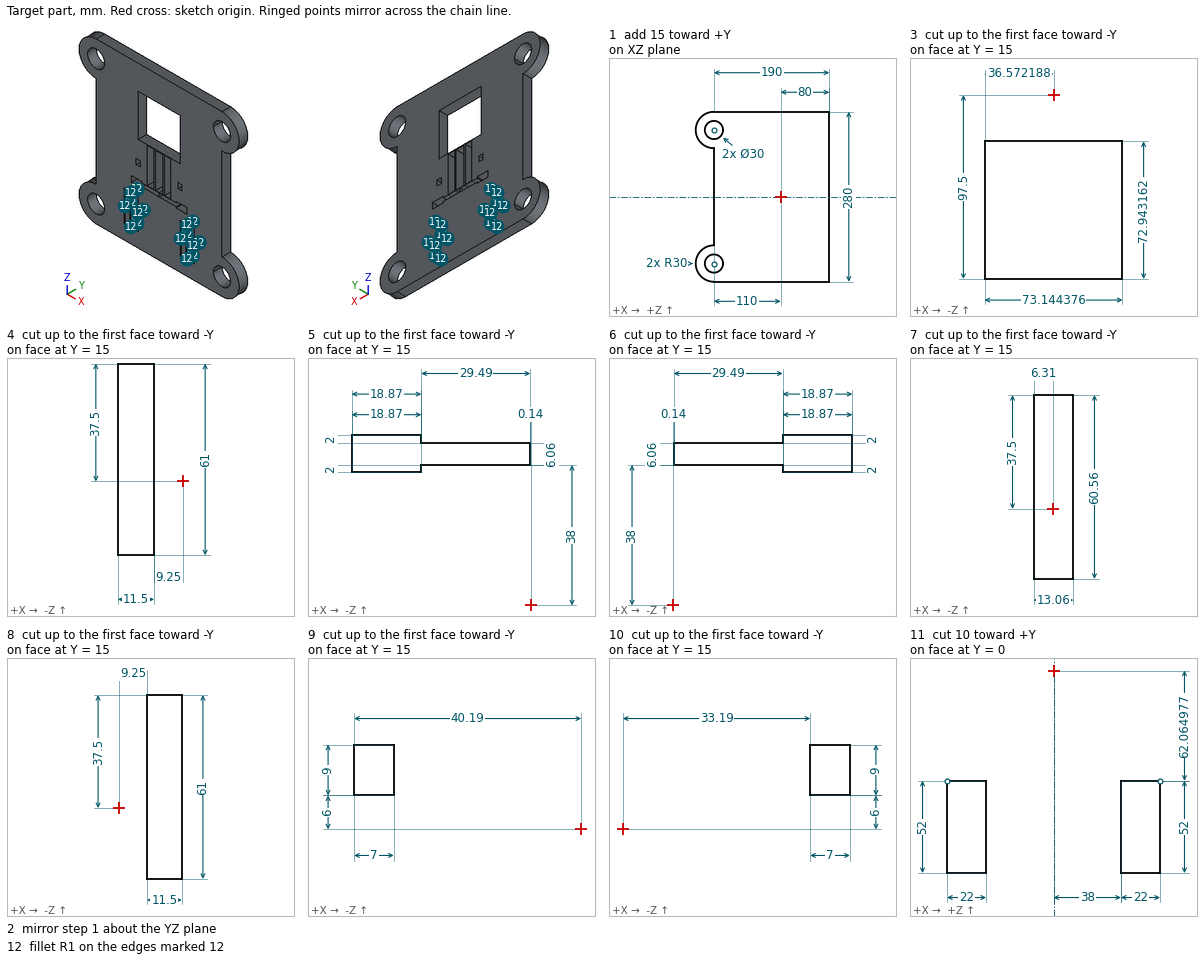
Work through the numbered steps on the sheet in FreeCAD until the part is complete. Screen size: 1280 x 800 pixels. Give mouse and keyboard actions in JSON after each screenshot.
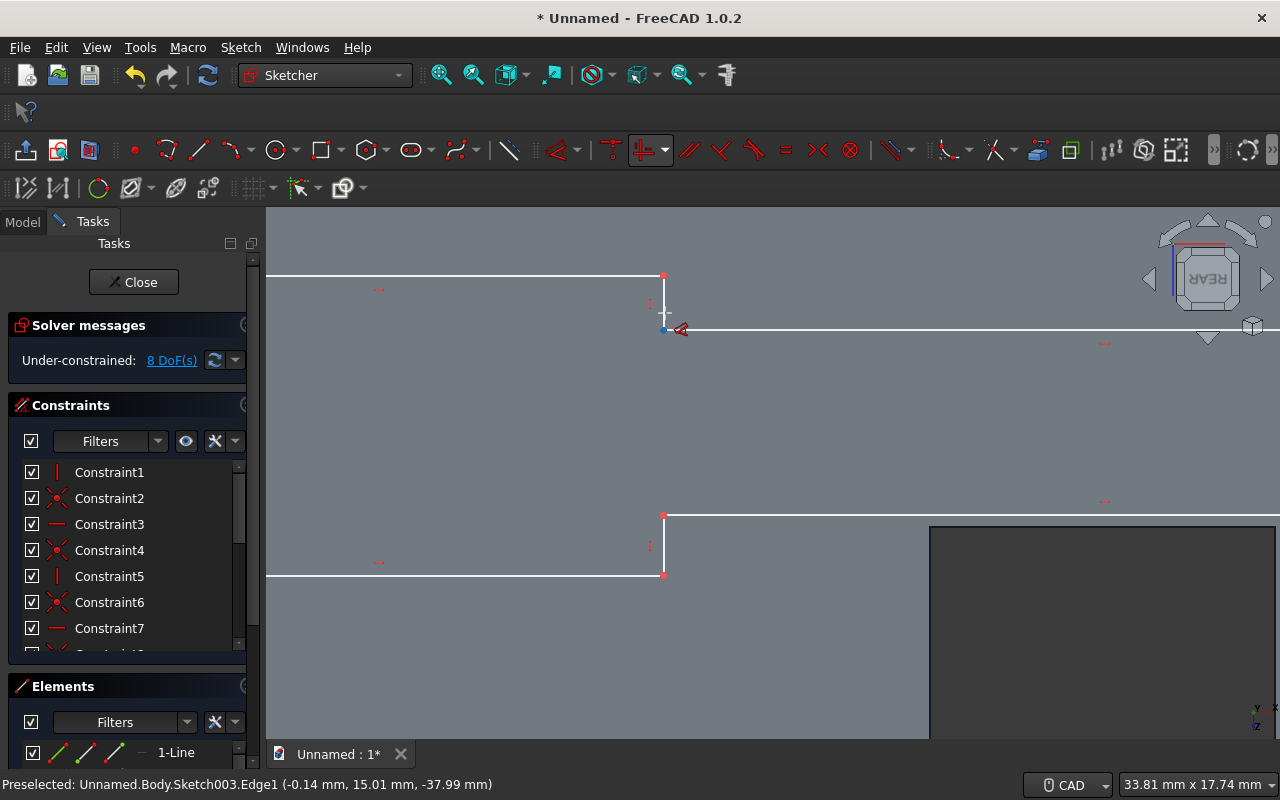
{"action": "left_click", "coordinate": [664, 314]}
{"action": "left_click", "coordinate": [630, 303]}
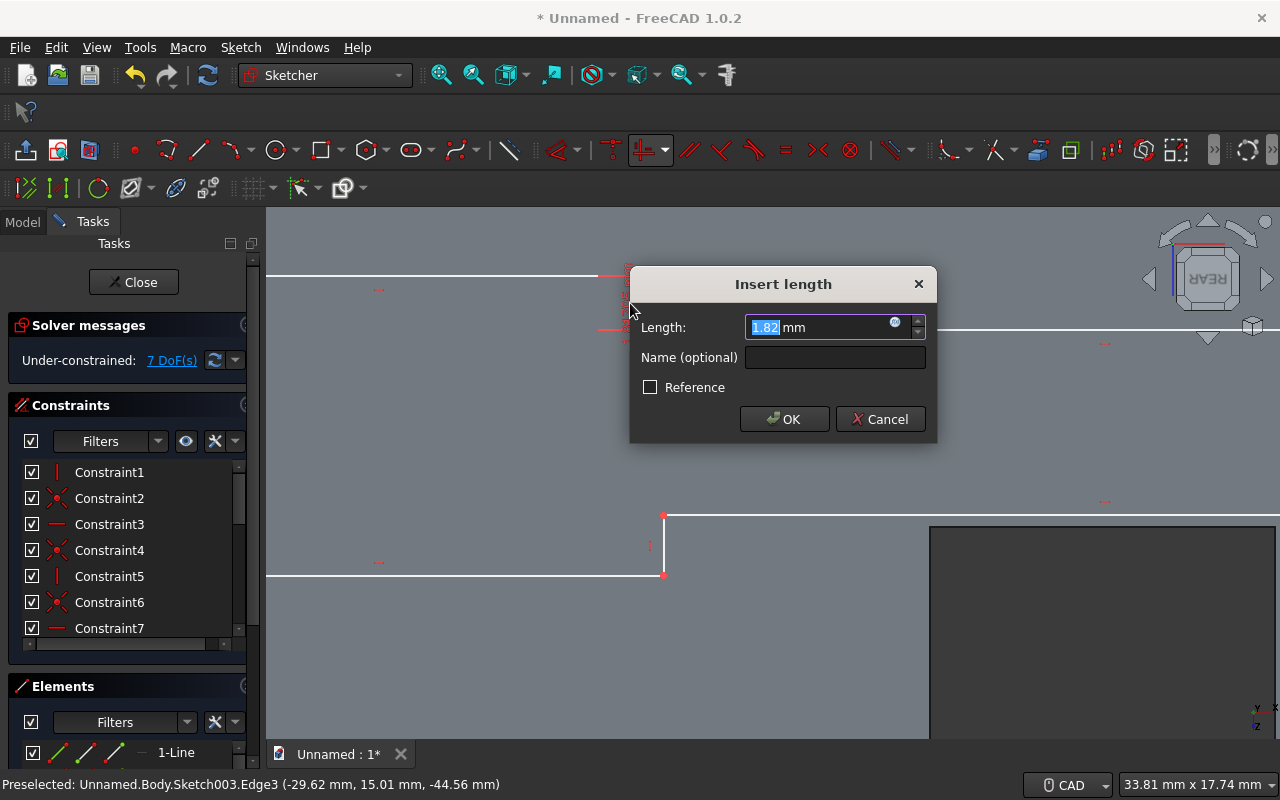
{"action": "type", "text": "2"}
{"action": "key", "text": "Return"}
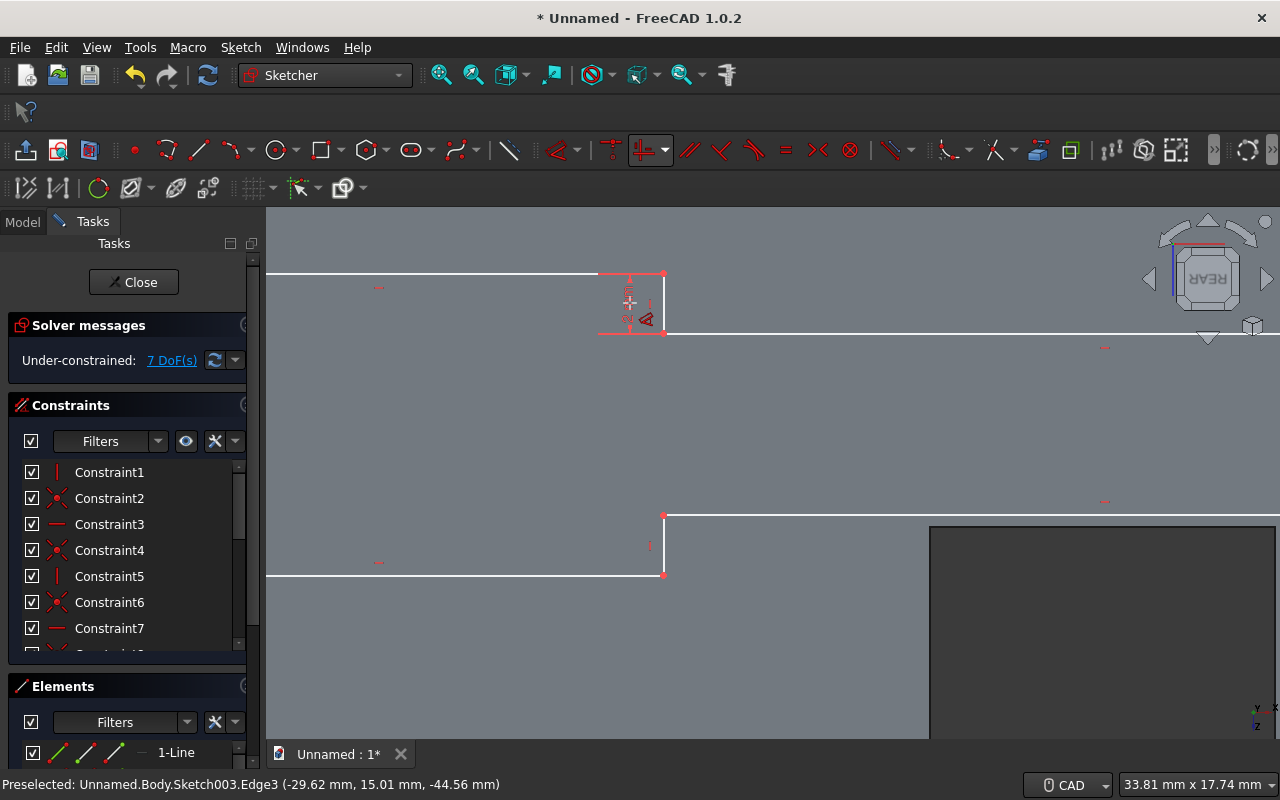
{"action": "left_click", "coordinate": [664, 558]}
{"action": "left_click", "coordinate": [630, 546]}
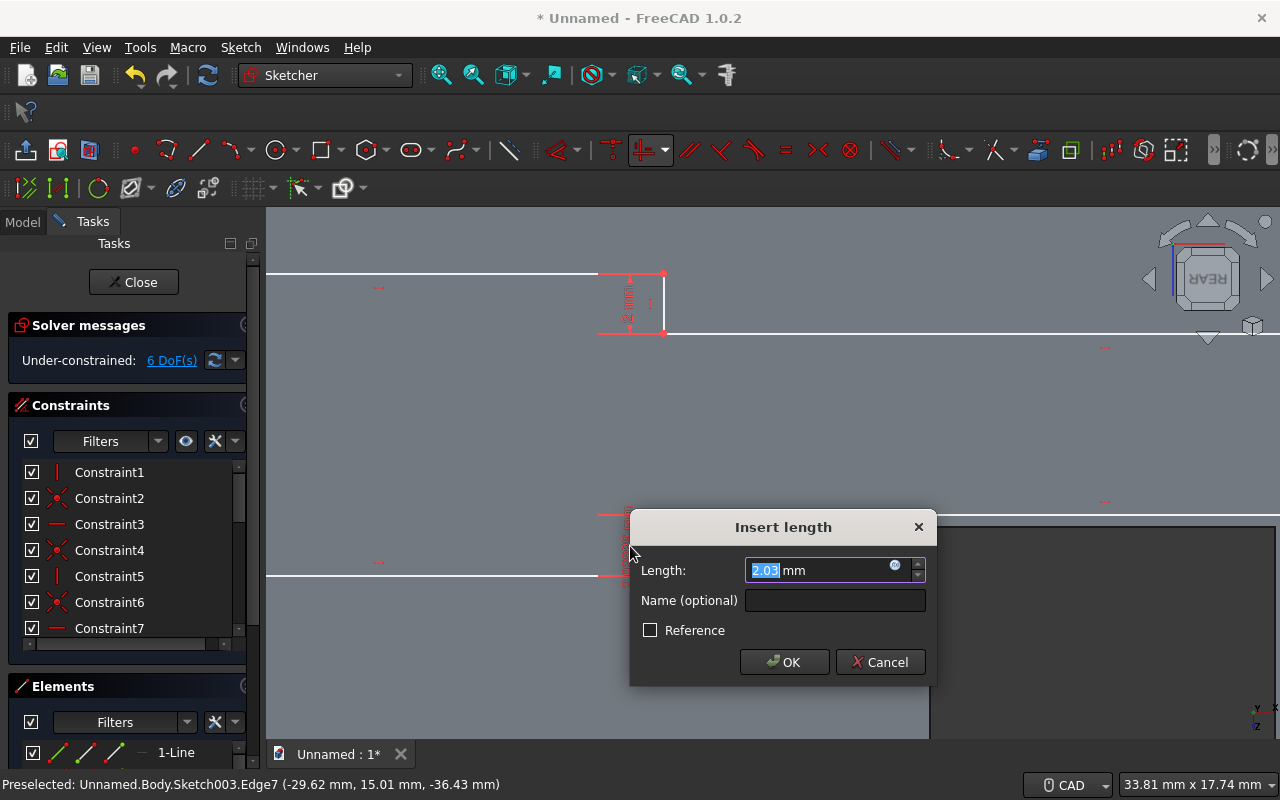
{"action": "type", "text": "2"}
{"action": "key", "text": "Return"}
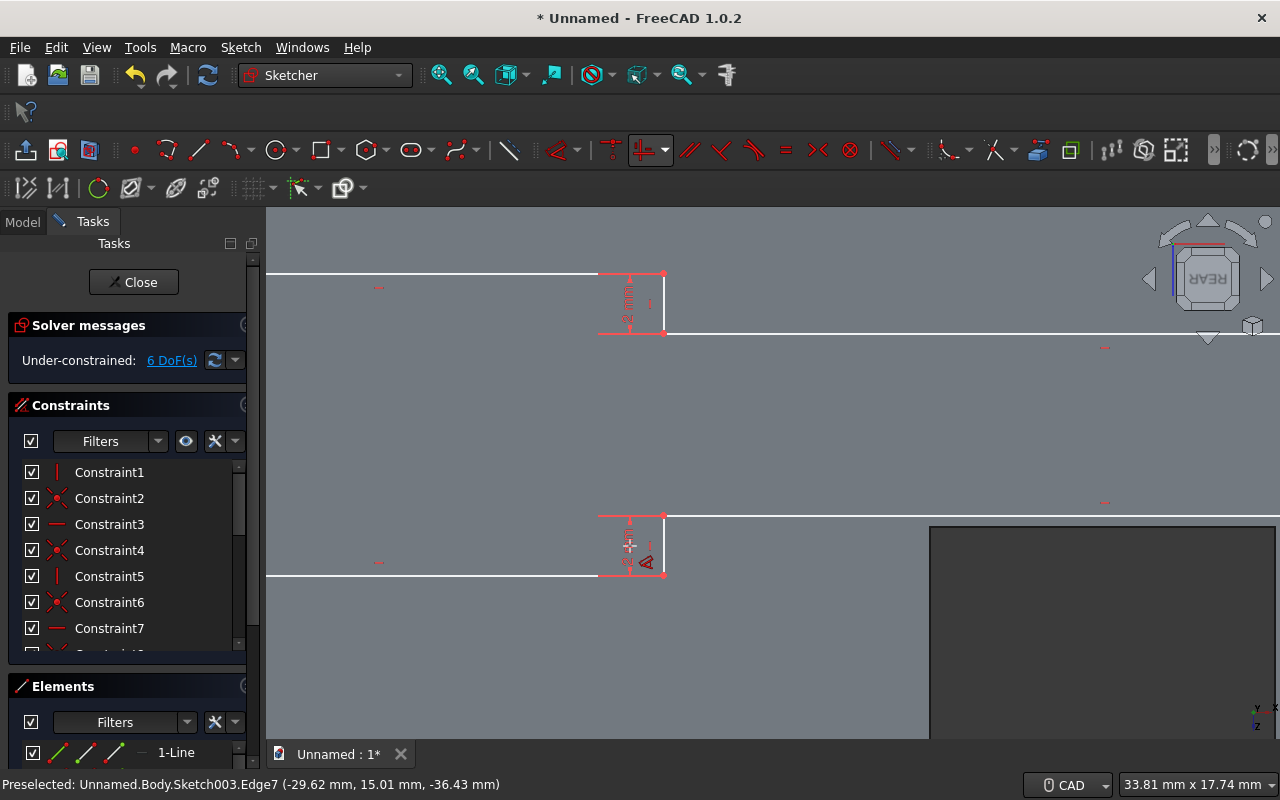
{"action": "scroll", "coordinate": [665, 313], "scroll_direction": "down", "scroll_amount": 7}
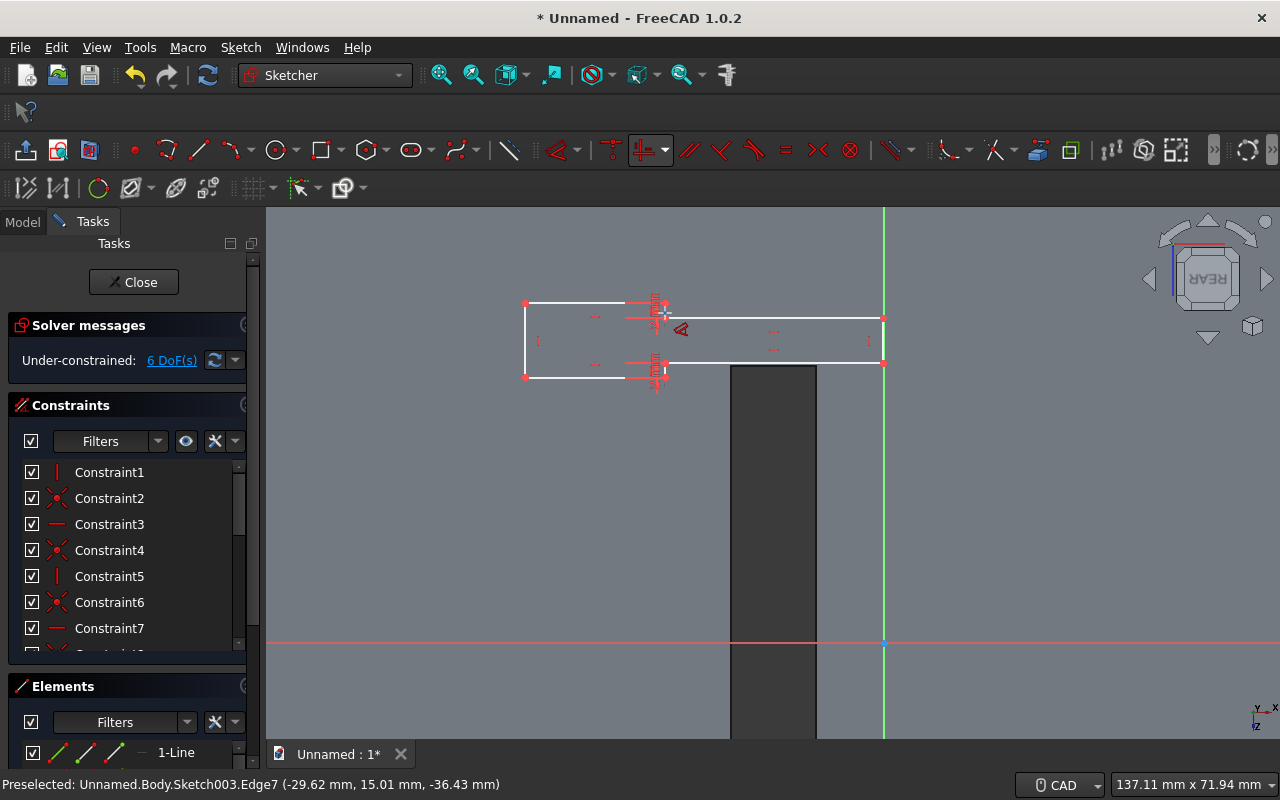
{"action": "left_click", "coordinate": [883, 363]}
{"action": "left_click", "coordinate": [918, 503]}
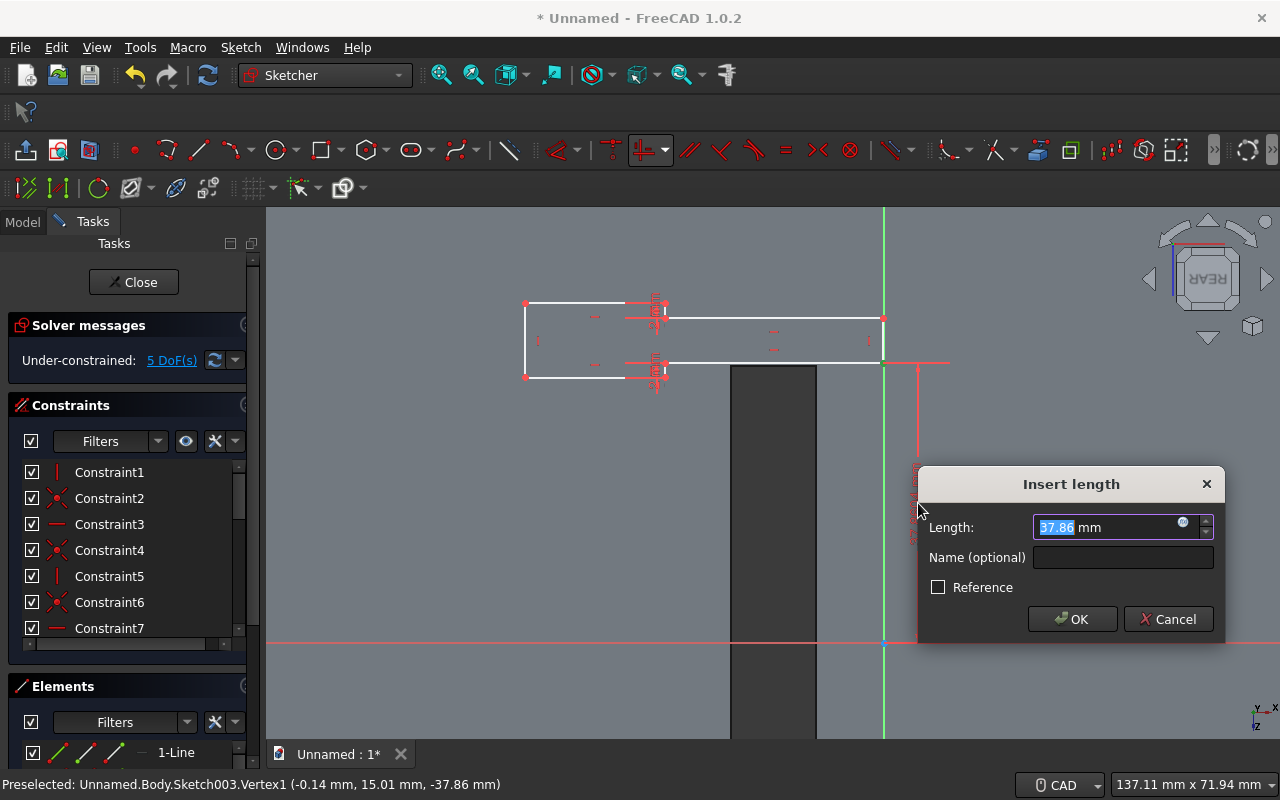
{"action": "type", "text": "38"}
{"action": "key", "text": "Return"}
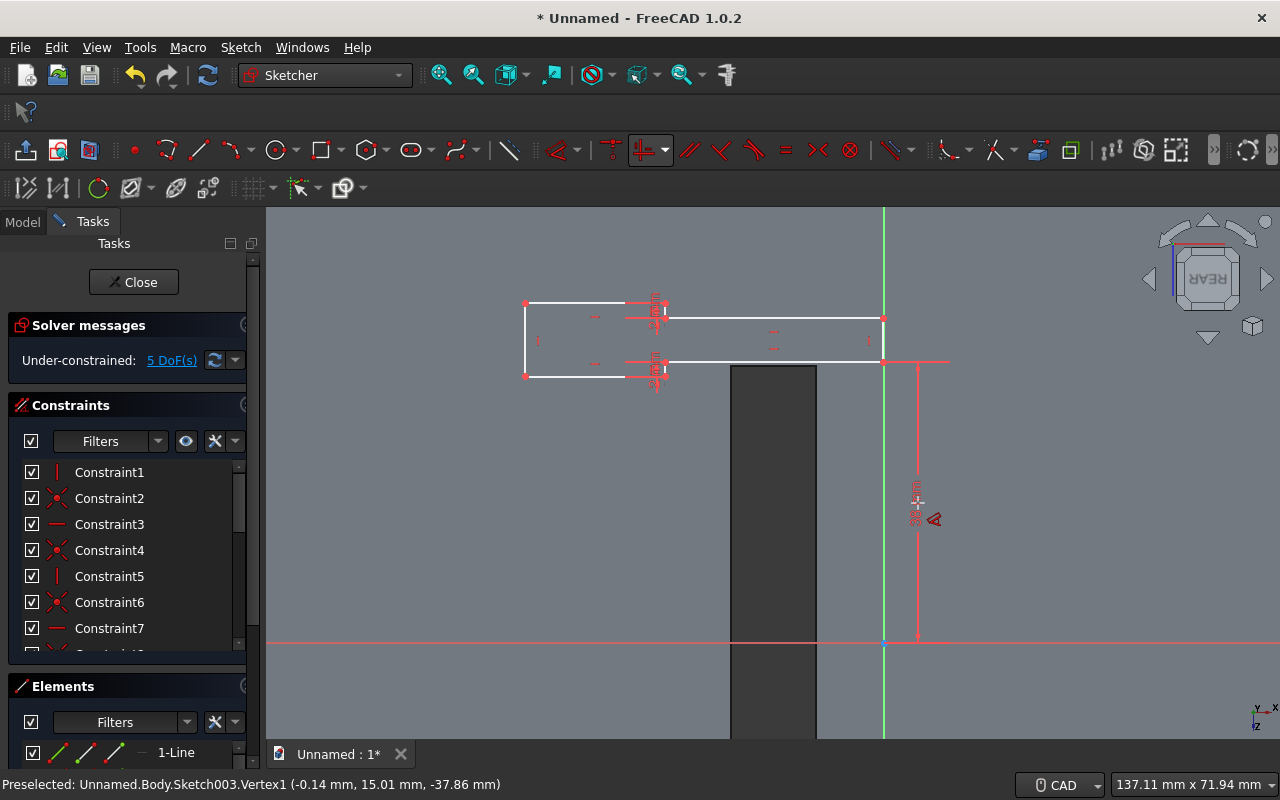
{"action": "left_click", "coordinate": [883, 349]}
{"action": "left_click", "coordinate": [917, 340]}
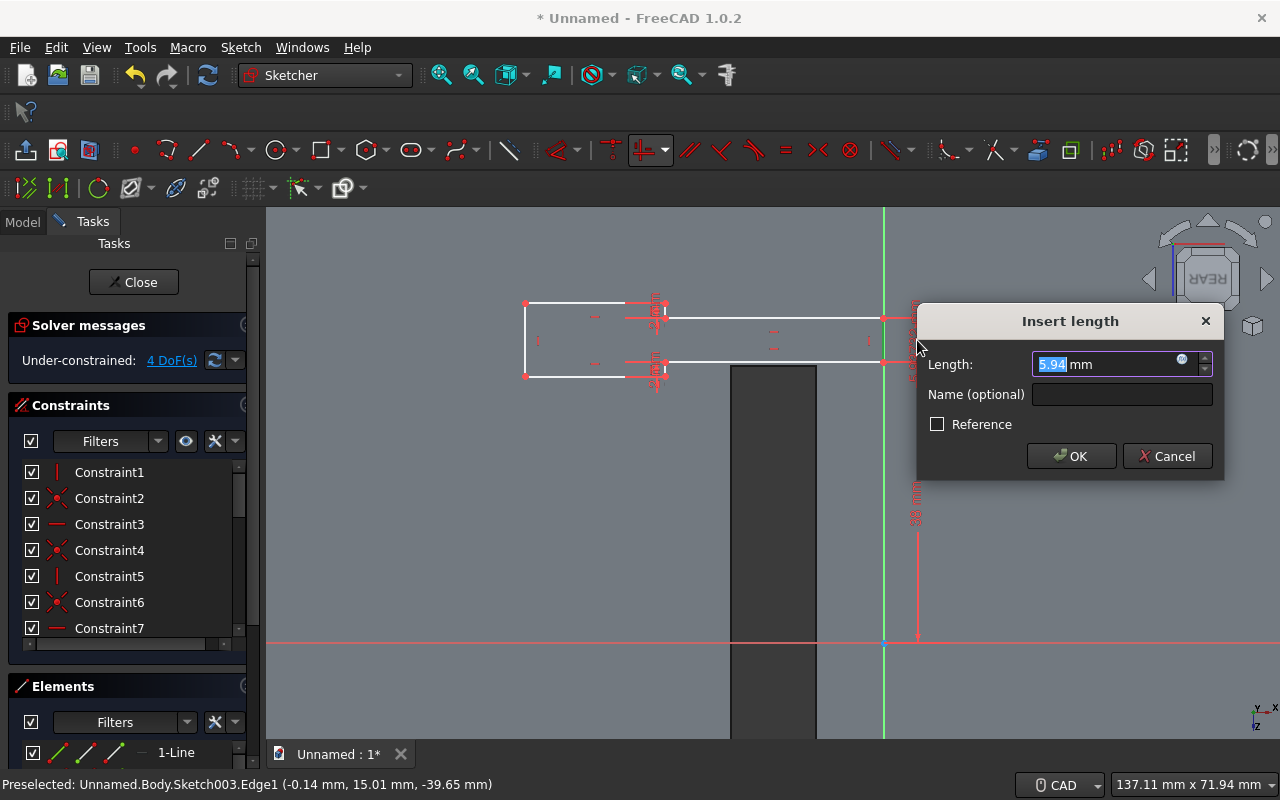
{"action": "type", "text": "6.06"}
{"action": "key", "text": "Return"}